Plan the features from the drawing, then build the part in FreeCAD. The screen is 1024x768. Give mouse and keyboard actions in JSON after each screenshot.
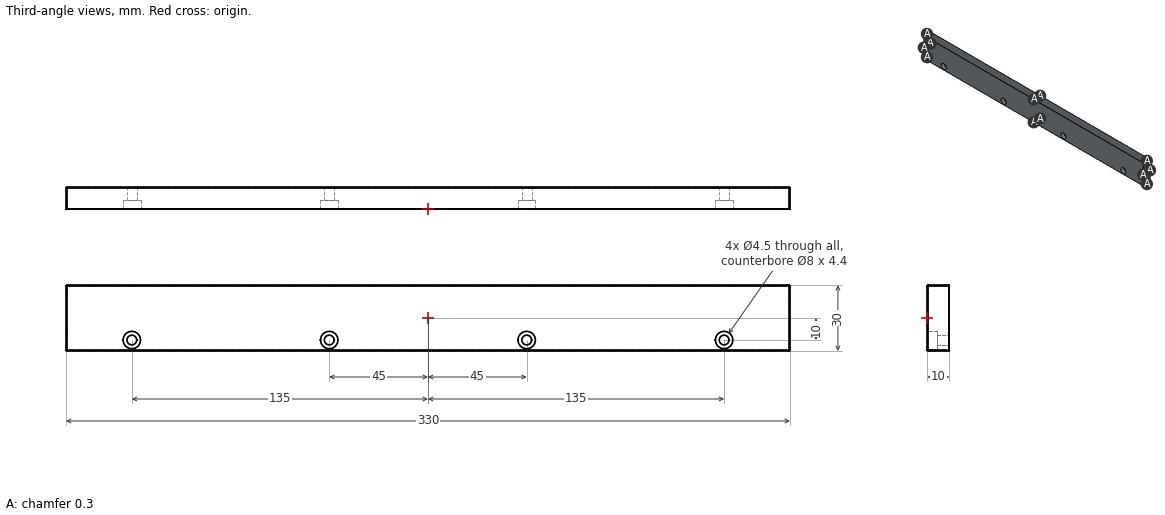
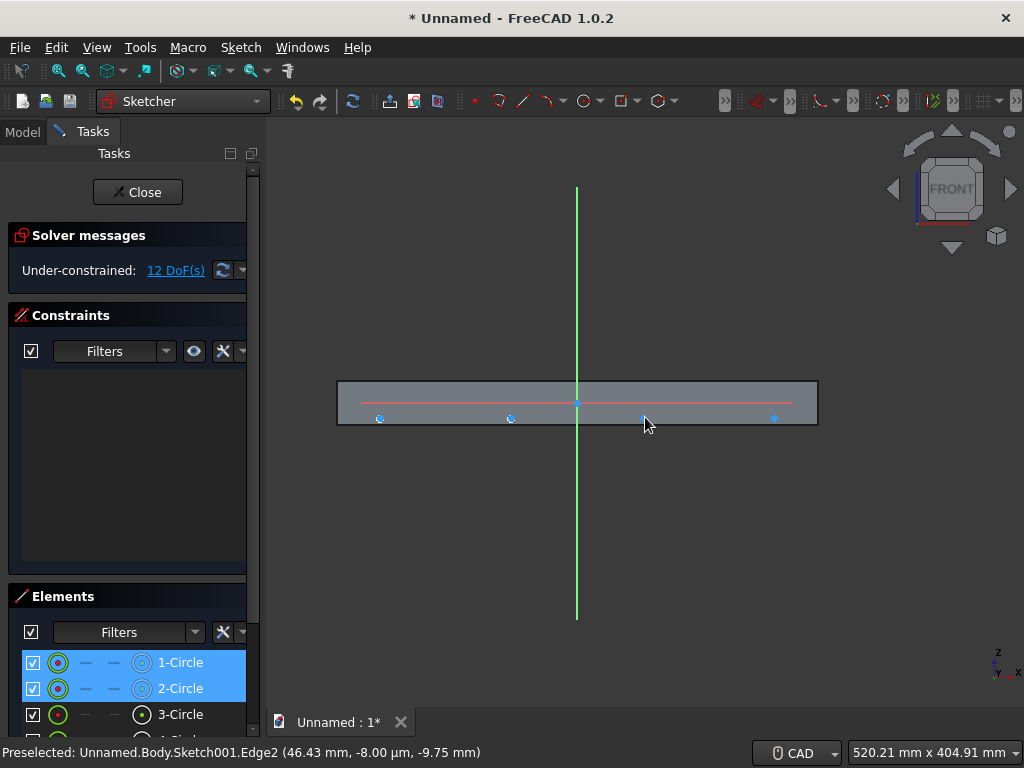
{"action": "scroll", "coordinate": [513, 417], "scroll_direction": "up", "scroll_amount": 8}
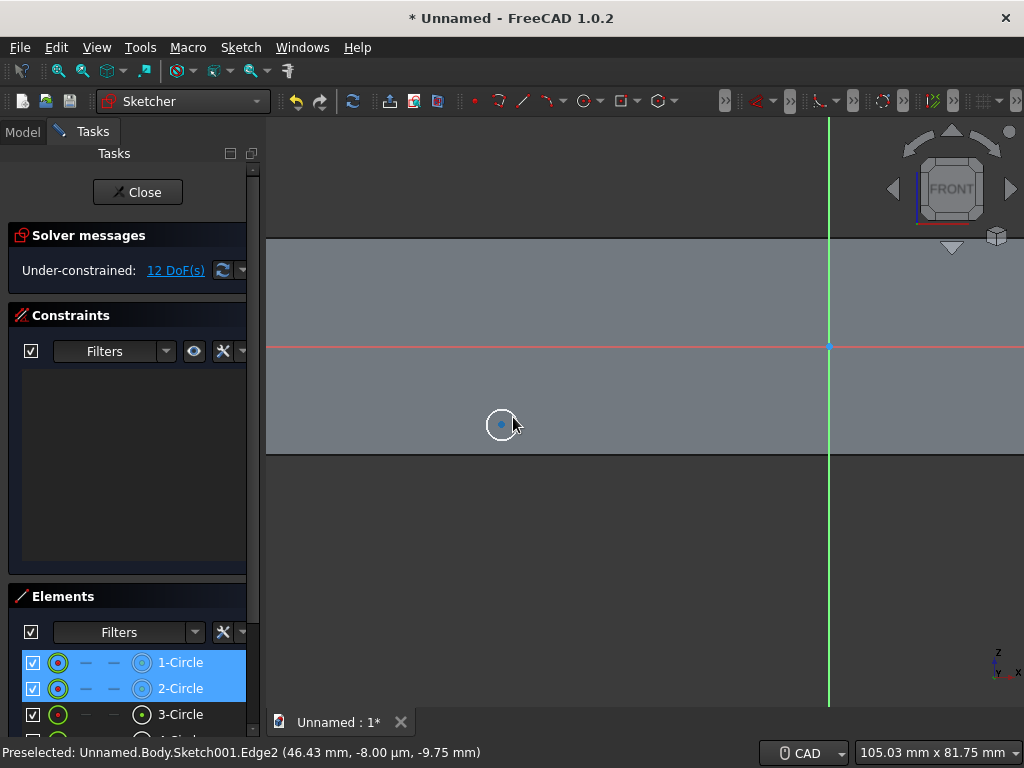
{"action": "left_click", "coordinate": [513, 414]}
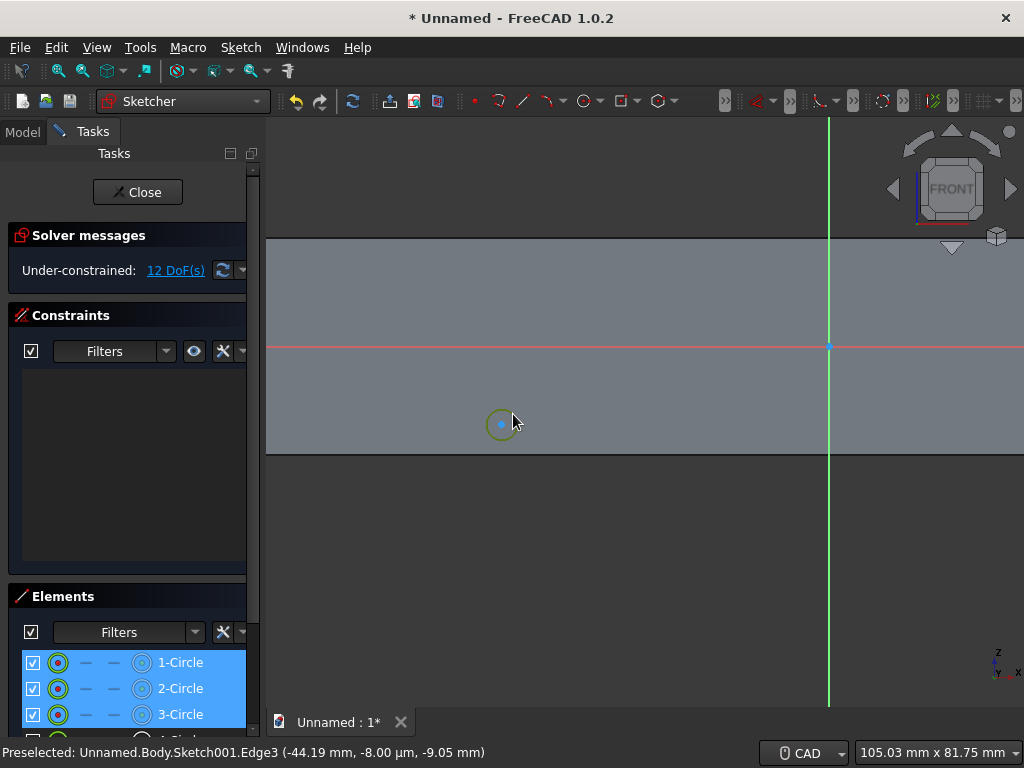
{"action": "scroll", "coordinate": [513, 417], "scroll_direction": "down", "scroll_amount": 8}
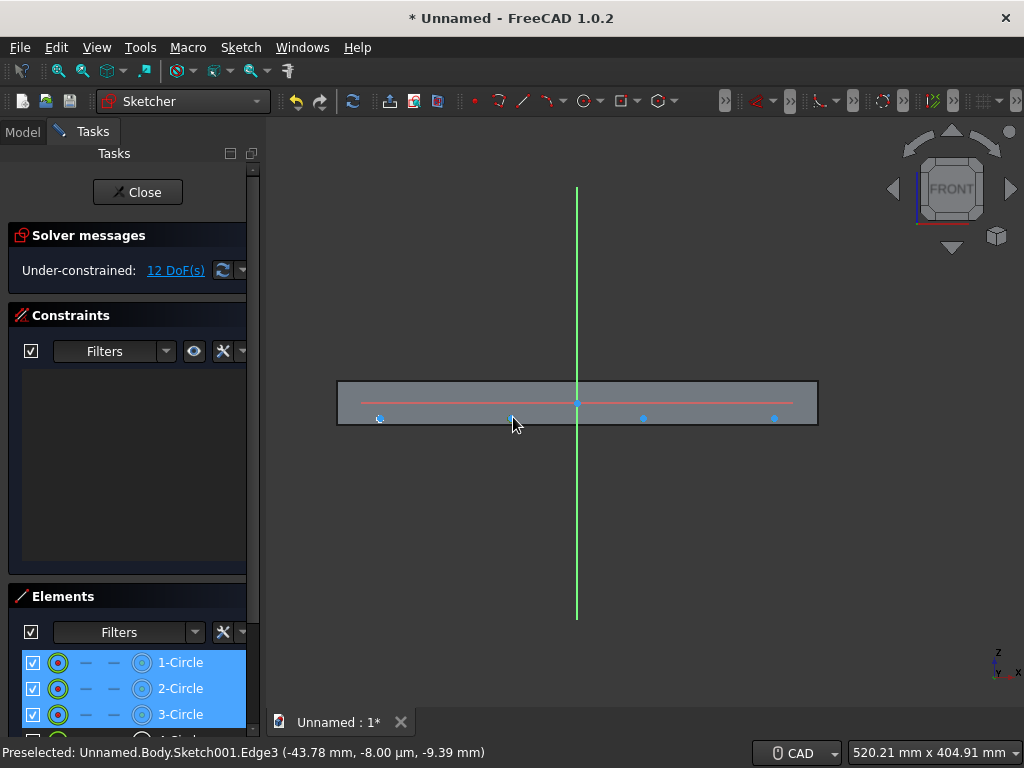
{"action": "scroll", "coordinate": [382, 417], "scroll_direction": "up", "scroll_amount": 8}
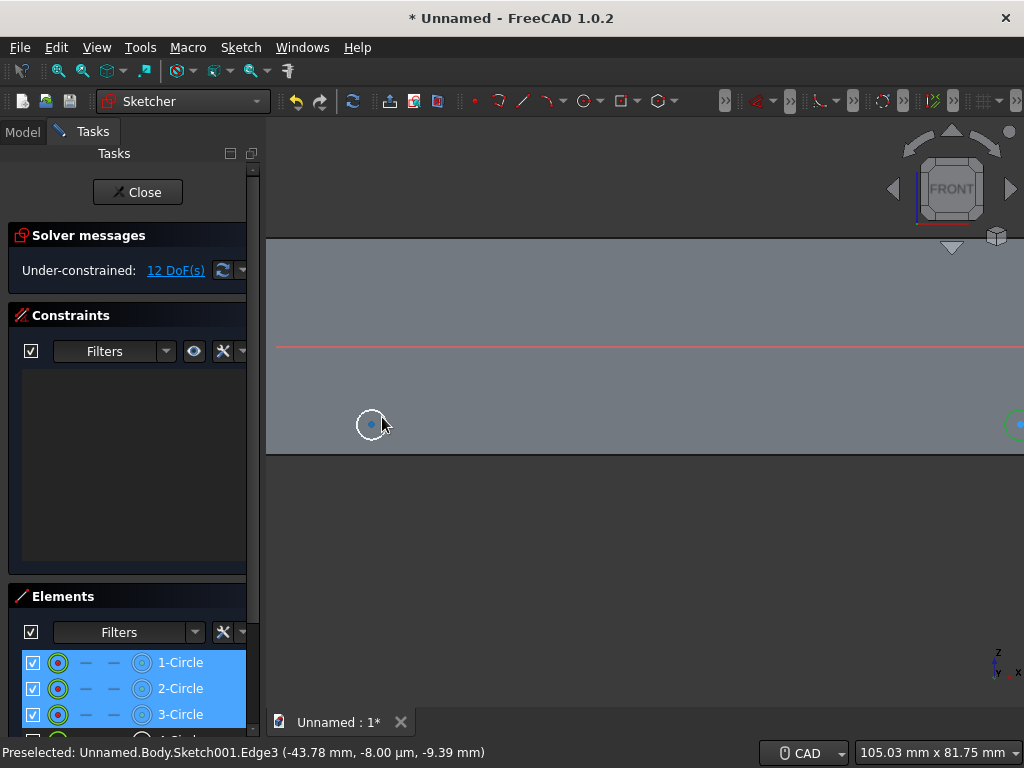
{"action": "left_click", "coordinate": [382, 414]}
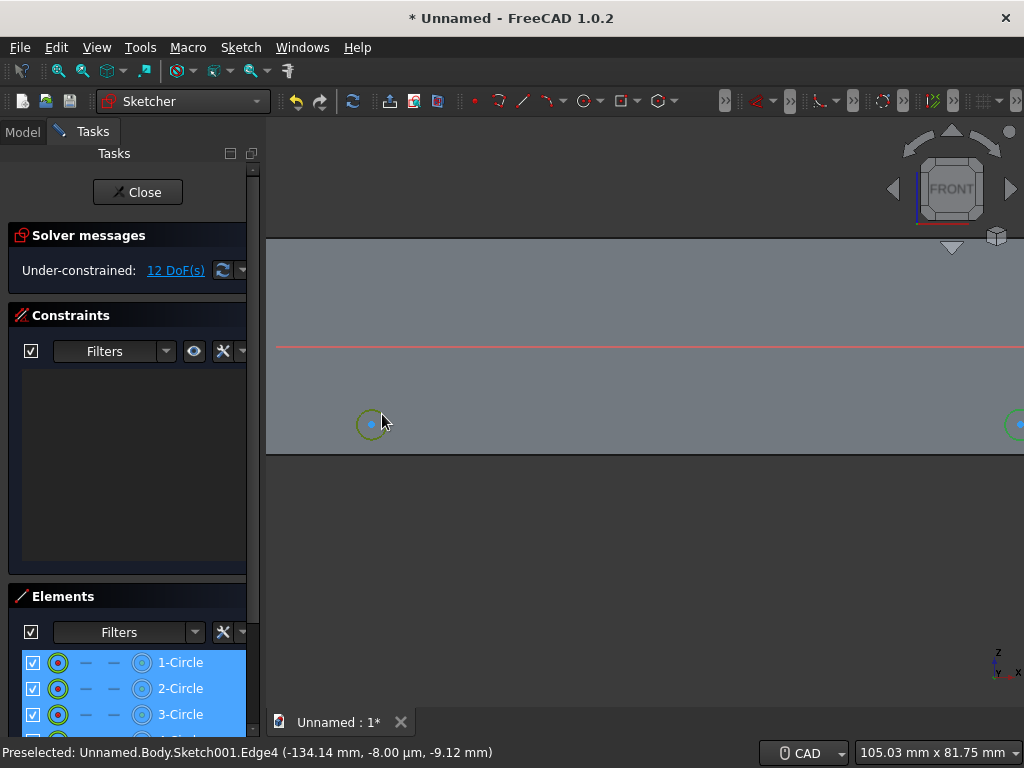
{"action": "key", "text": "e"}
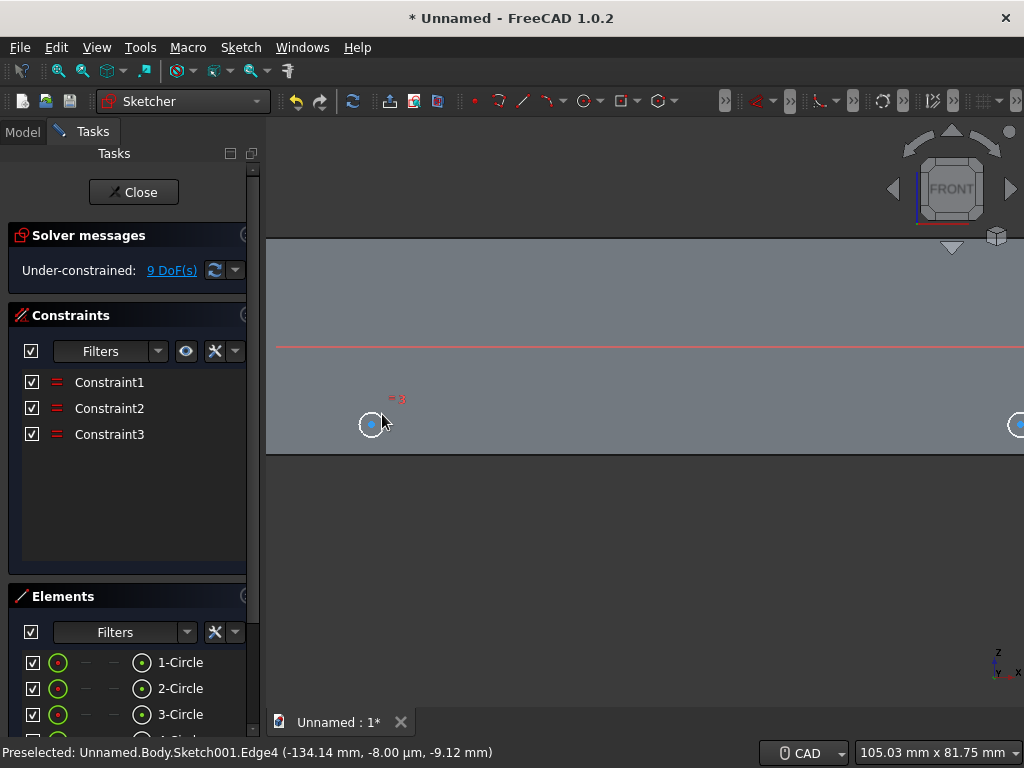
{"action": "scroll", "coordinate": [381, 417], "scroll_direction": "down", "scroll_amount": 8}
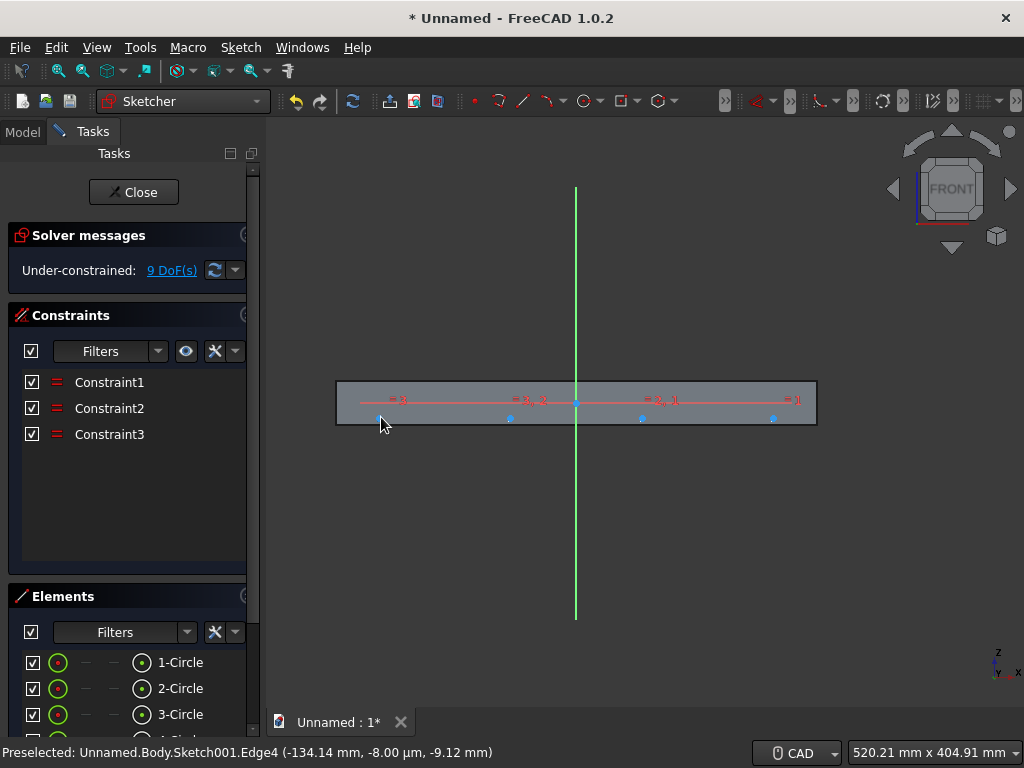
{"action": "left_click", "coordinate": [773, 419]}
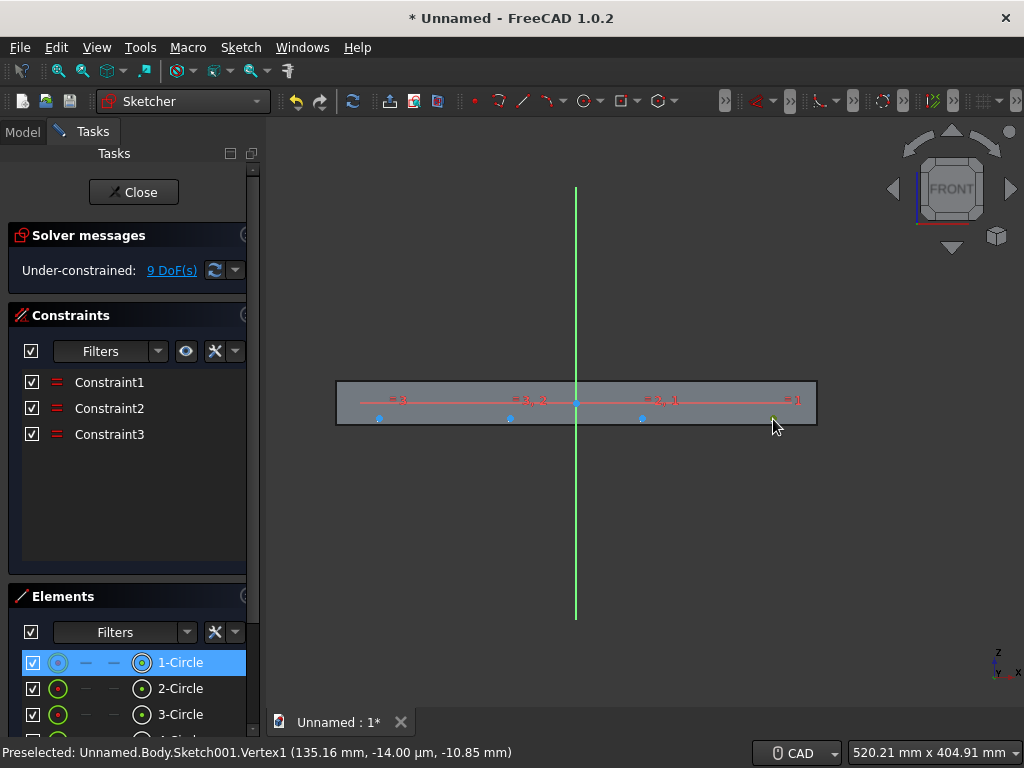
{"action": "left_click", "coordinate": [642, 419]}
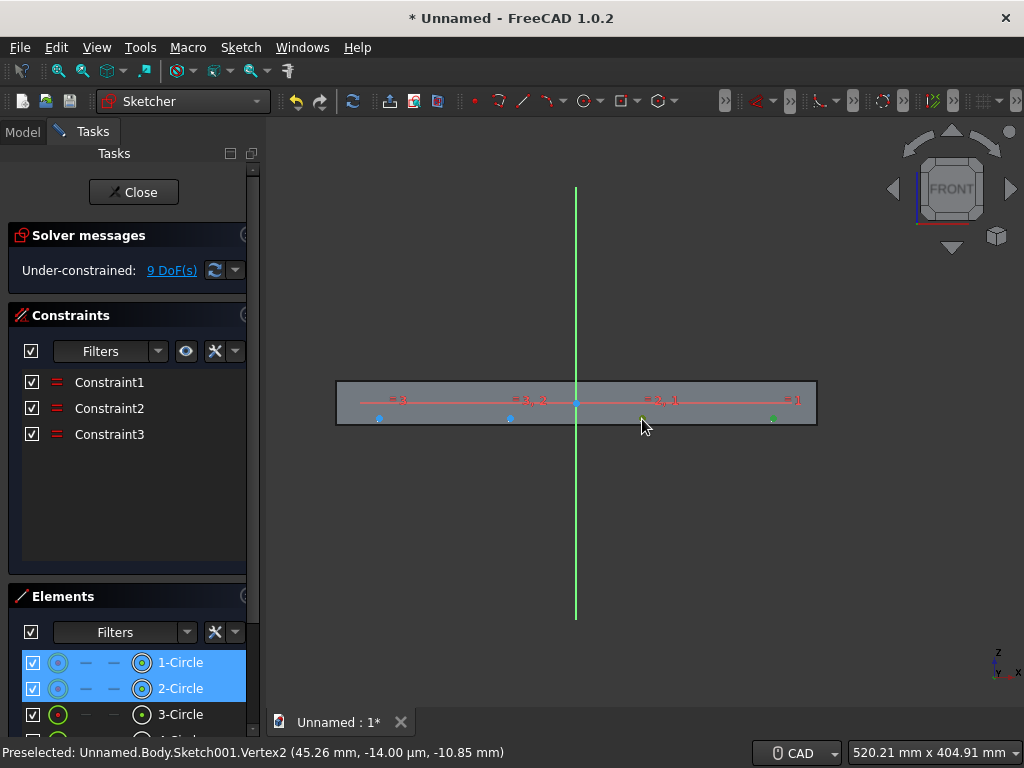
{"action": "key", "text": "h"}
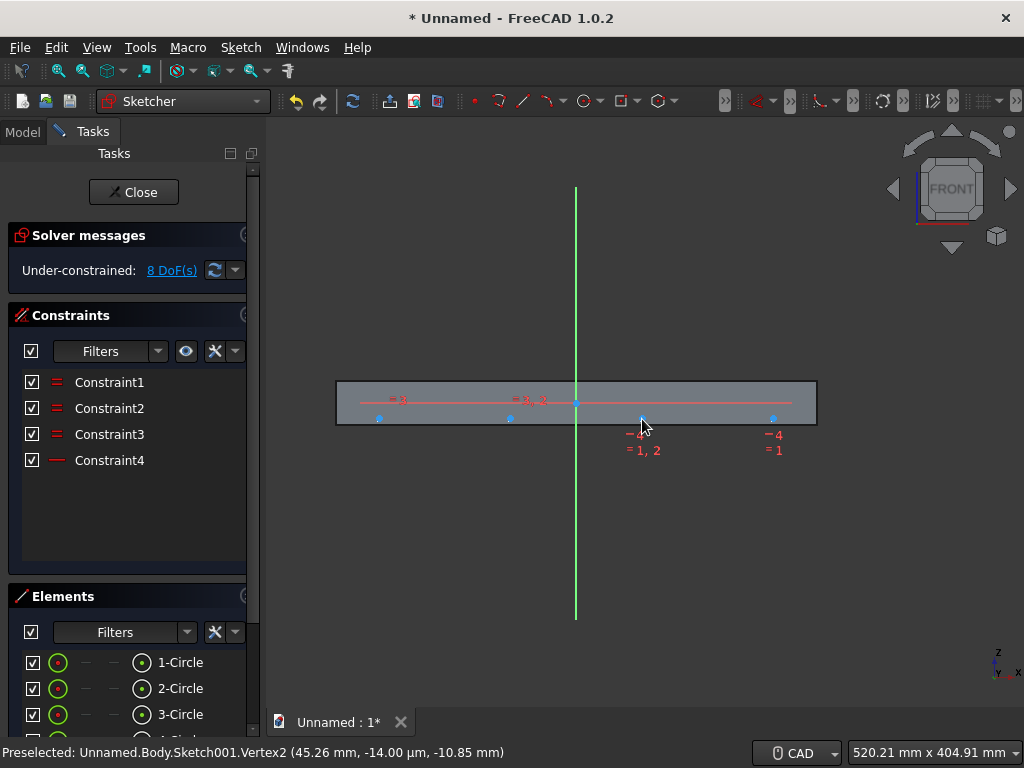
{"action": "left_click", "coordinate": [642, 419]}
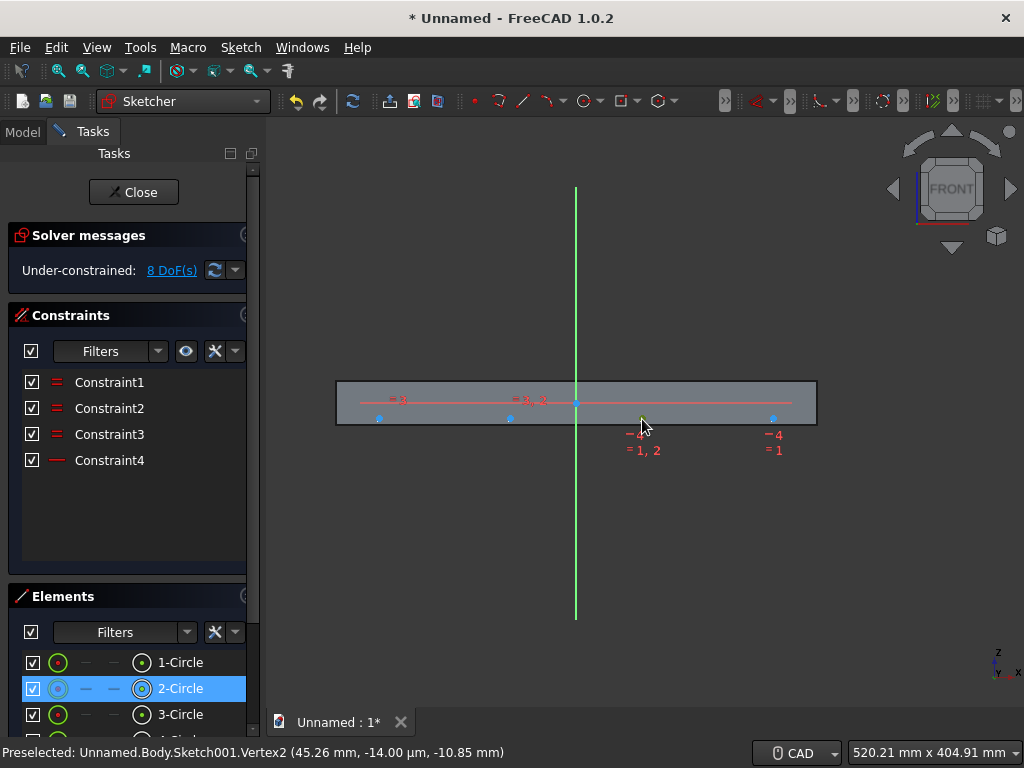
{"action": "left_click", "coordinate": [510, 419]}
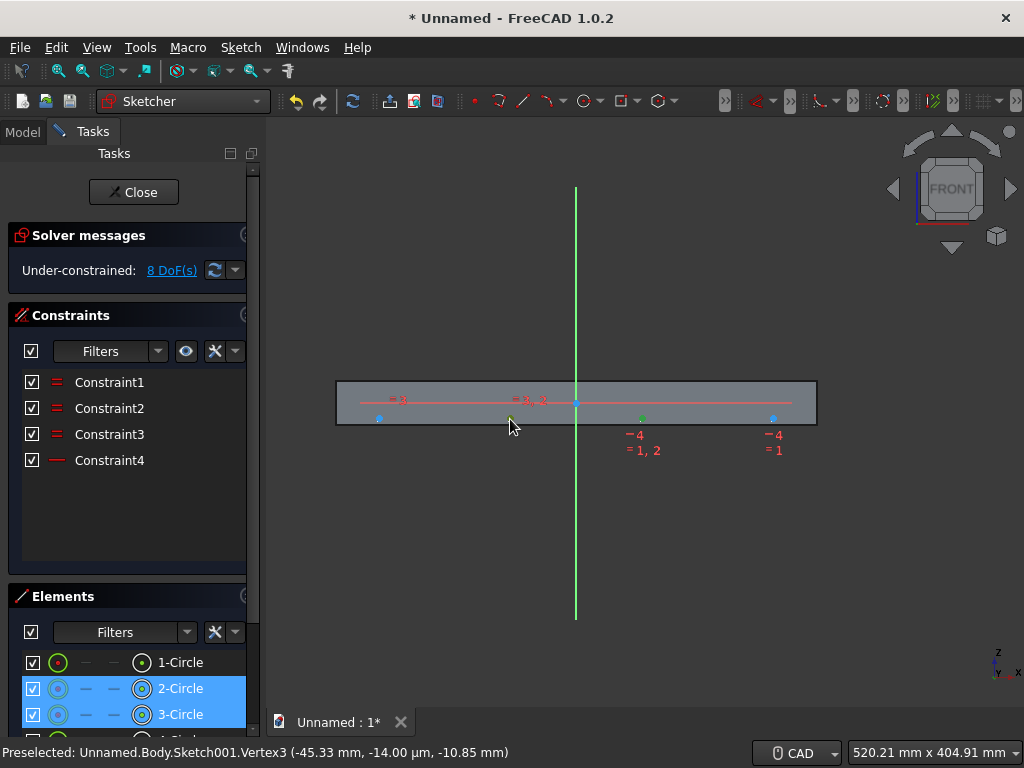
{"action": "key", "text": "h"}